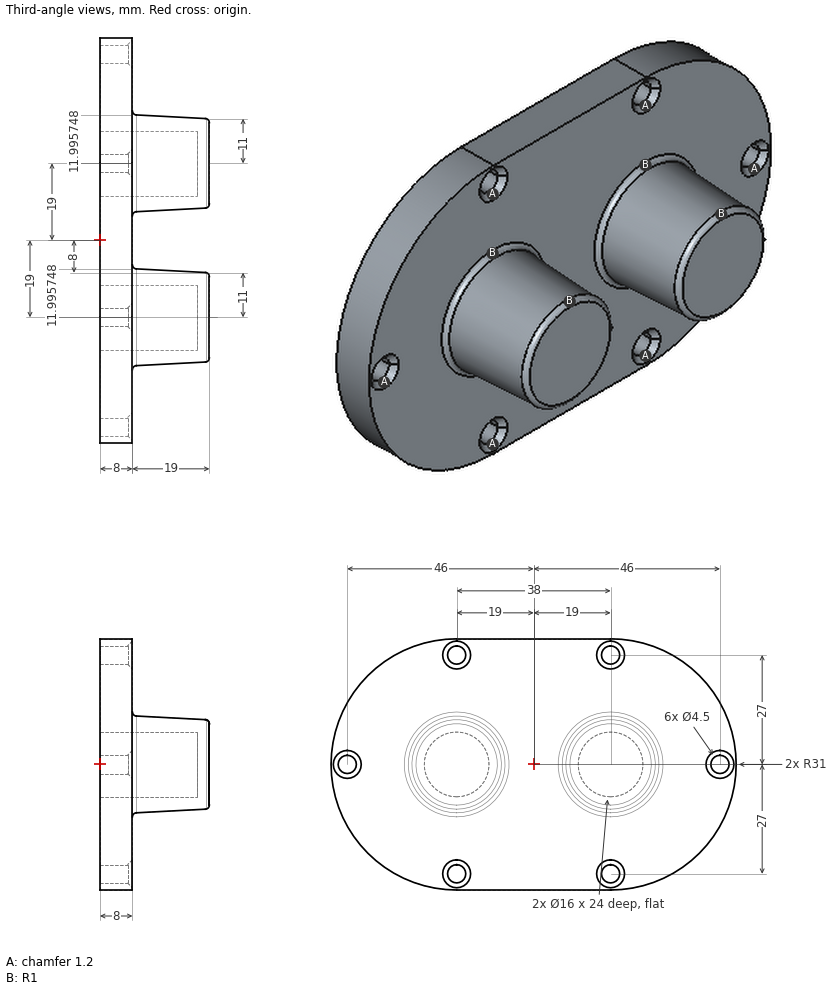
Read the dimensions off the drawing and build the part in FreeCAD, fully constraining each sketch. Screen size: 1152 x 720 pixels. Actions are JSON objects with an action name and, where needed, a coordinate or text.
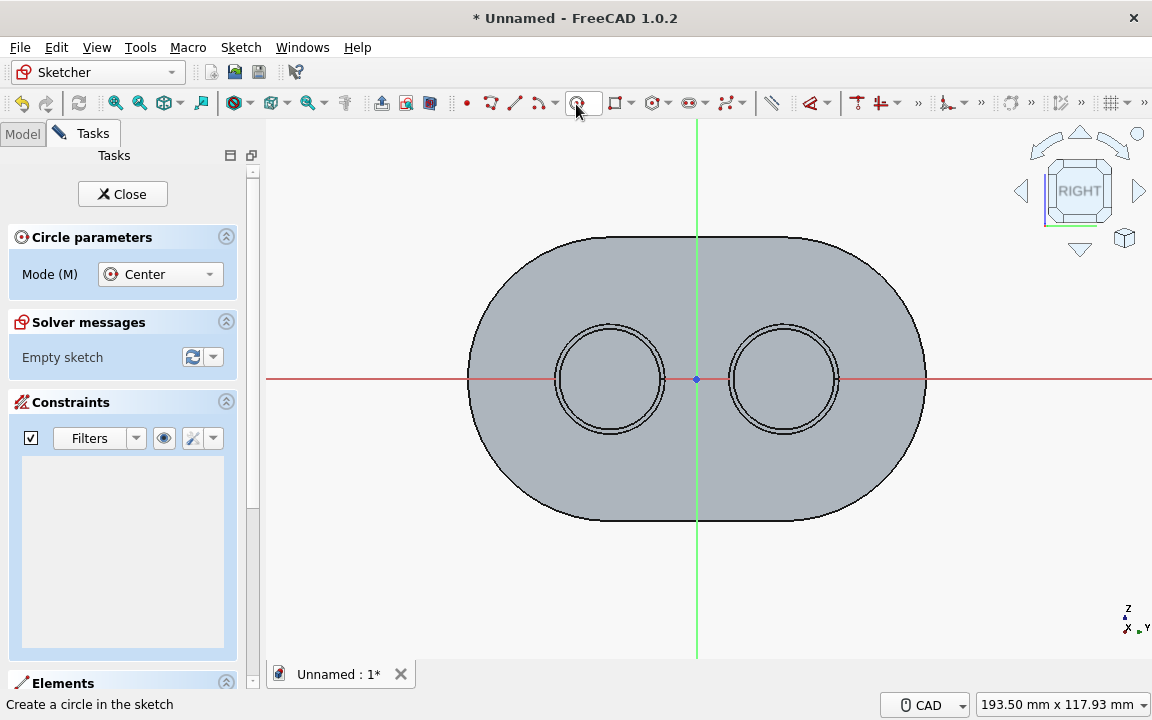
{"action": "scroll", "coordinate": [908, 379], "scroll_direction": "up", "scroll_amount": 4}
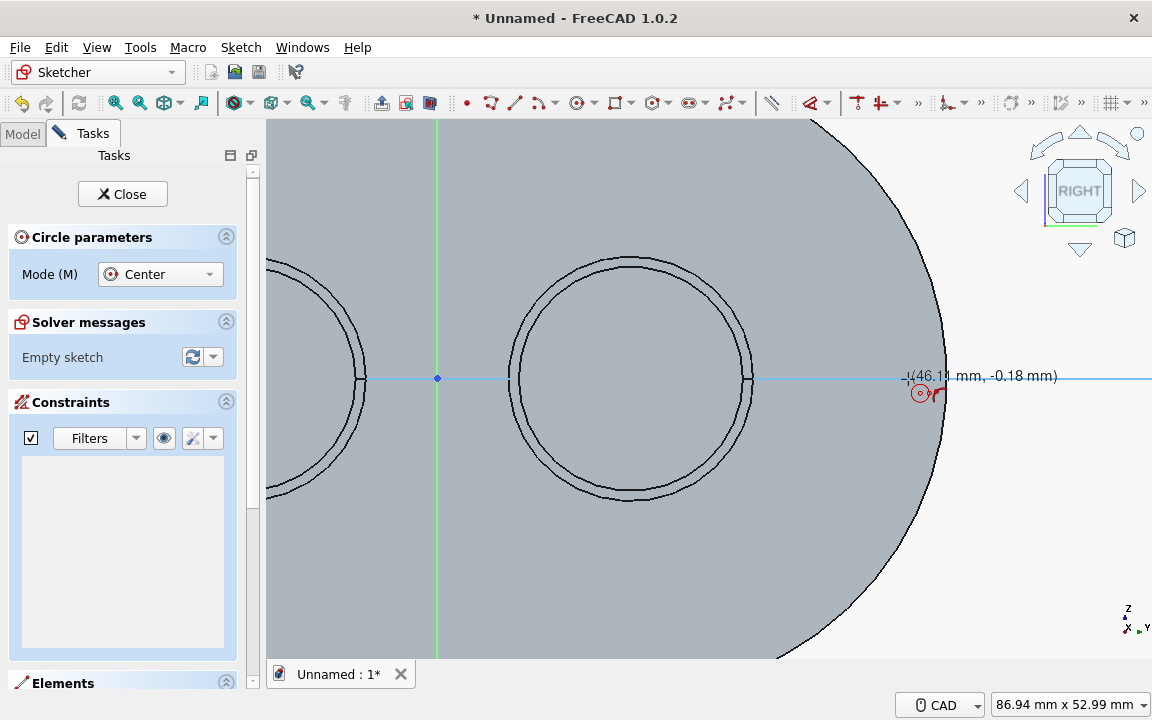
{"action": "left_click", "coordinate": [906, 379]}
{"action": "mouse_move", "coordinate": [922, 363]}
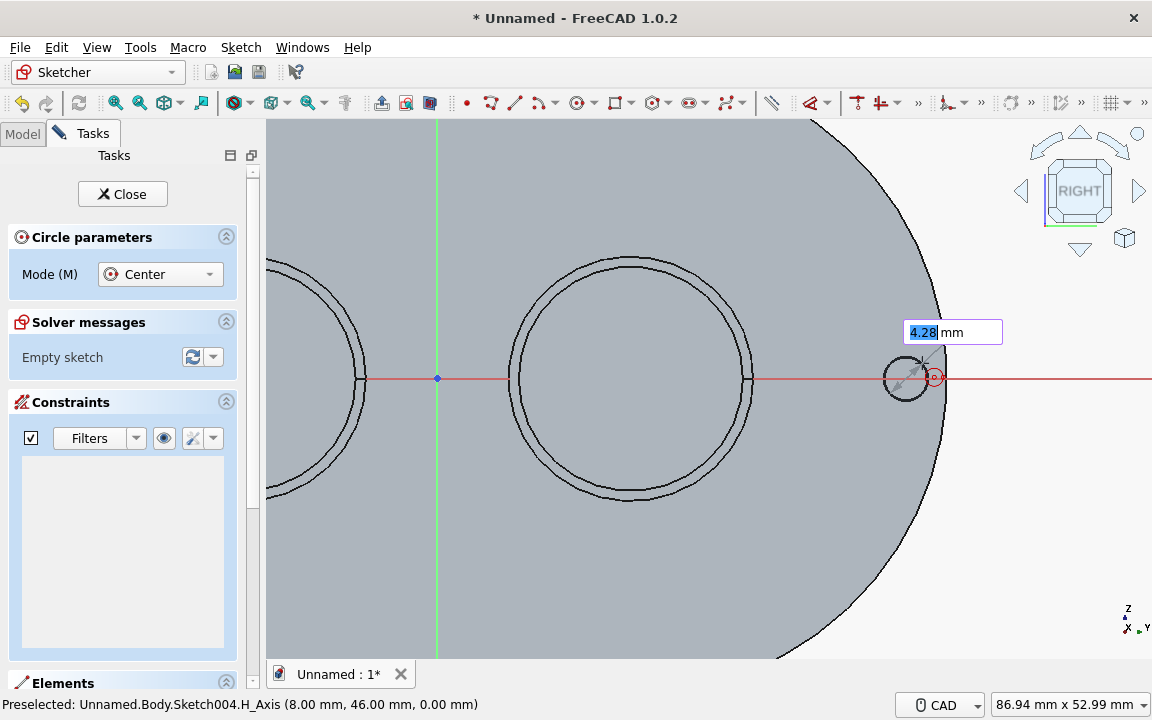
{"action": "type", "text": "4.5"}
{"action": "key", "text": "Return"}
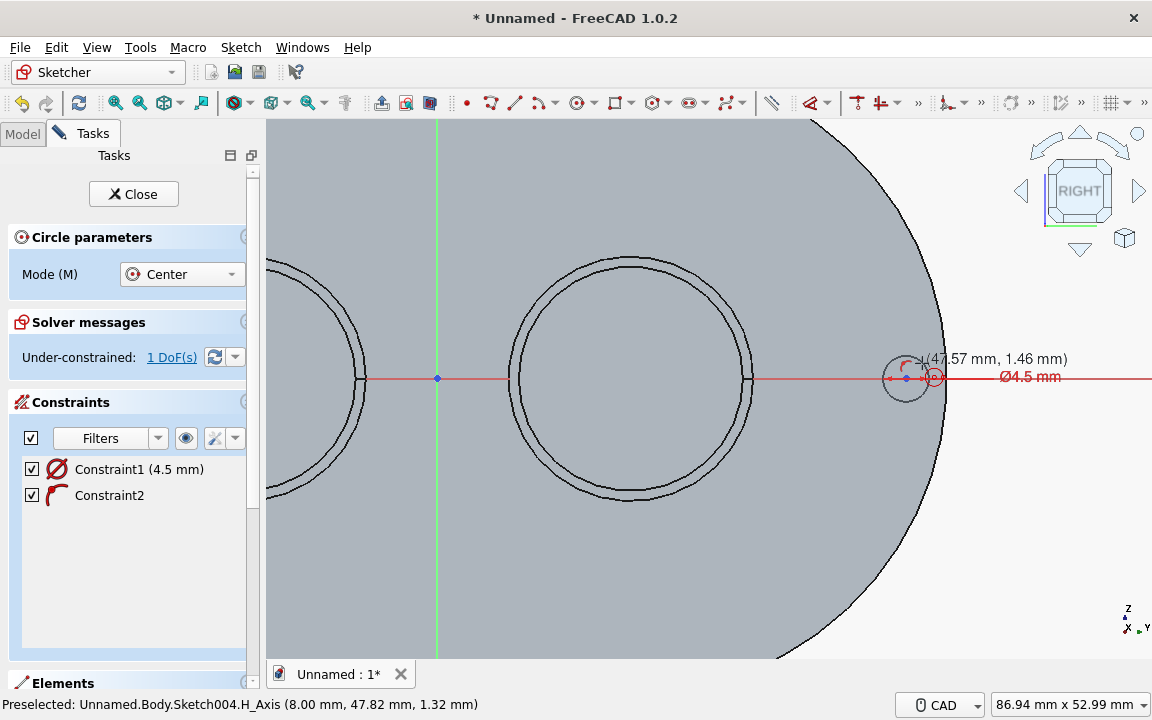
{"action": "scroll", "coordinate": [888, 401], "scroll_direction": "down", "scroll_amount": 3}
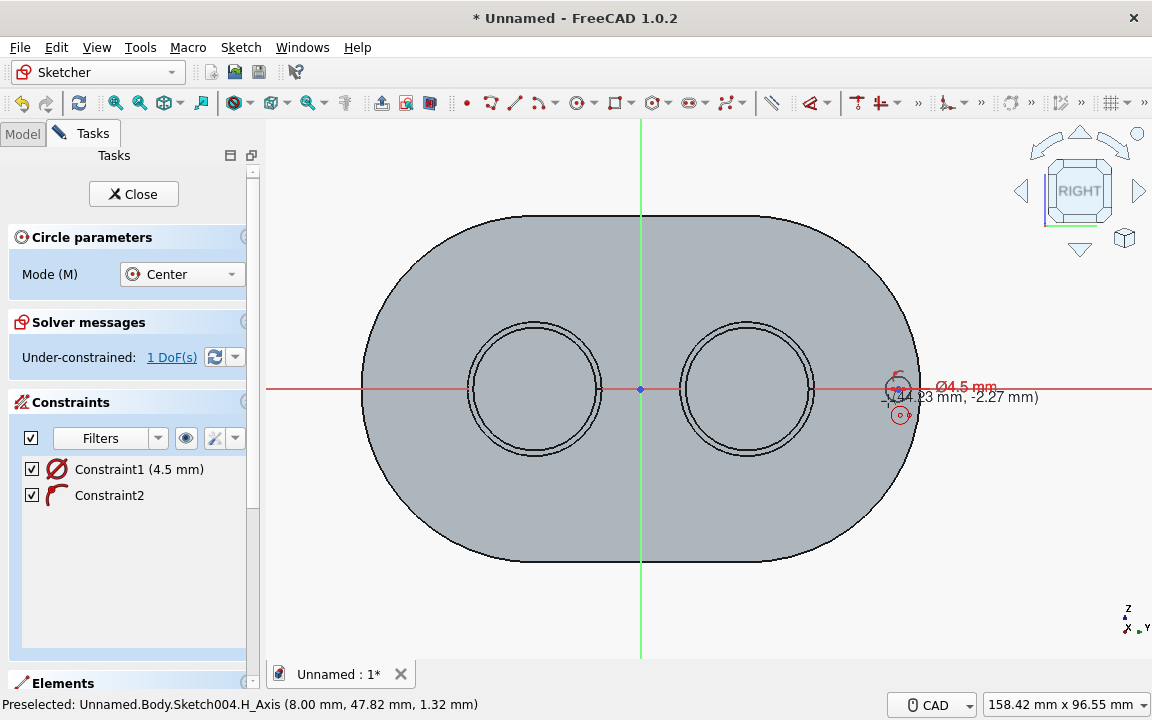
{"action": "scroll", "coordinate": [747, 238], "scroll_direction": "up", "scroll_amount": 3}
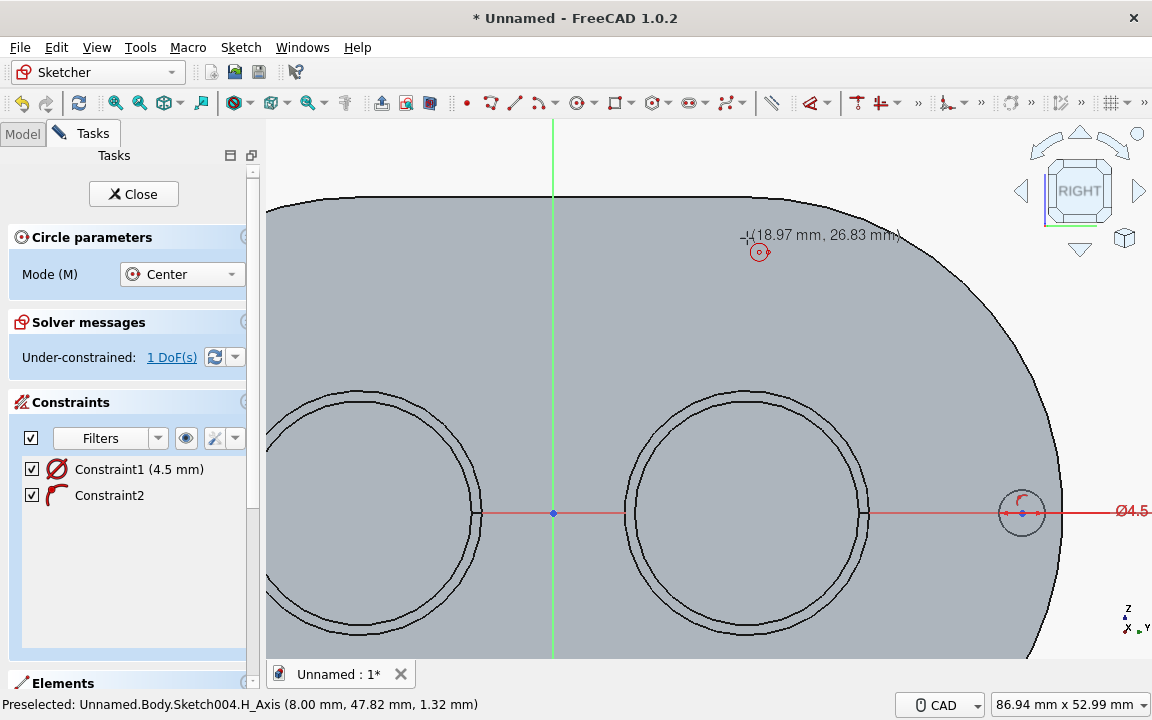
{"action": "left_click", "coordinate": [747, 238]}
{"action": "mouse_move", "coordinate": [763, 222]}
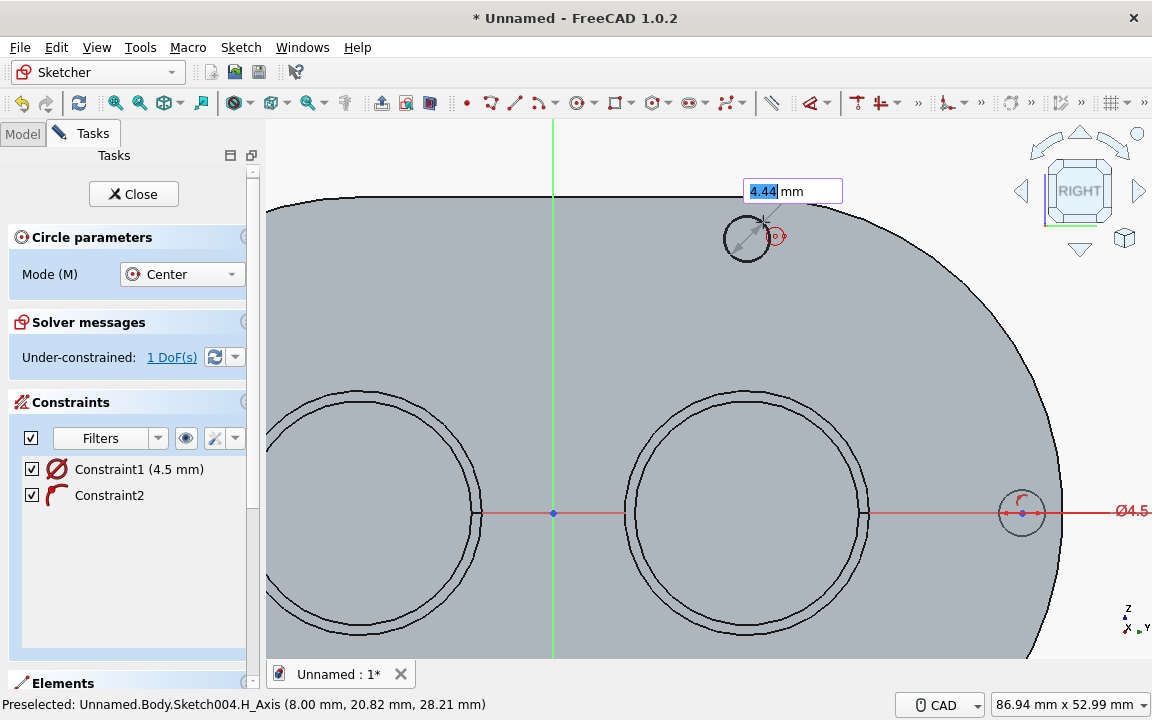
{"action": "type", "text": "4.5"}
{"action": "key", "text": "Return"}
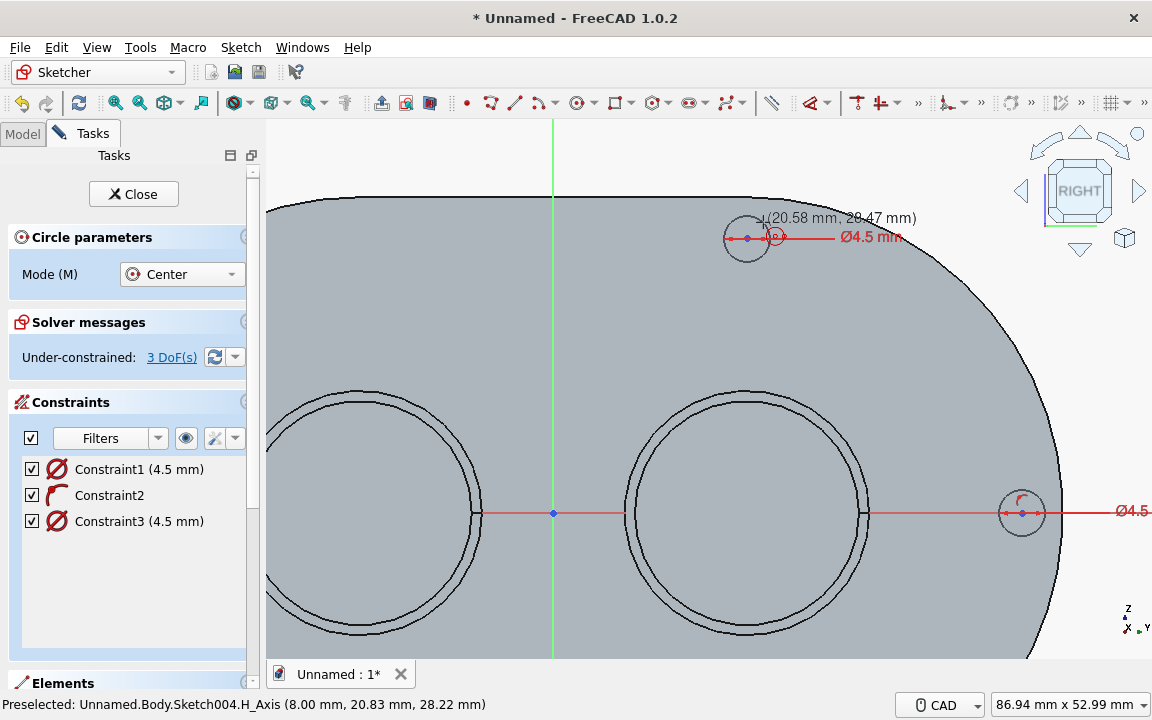
{"action": "scroll", "coordinate": [747, 238], "scroll_direction": "down", "scroll_amount": 3}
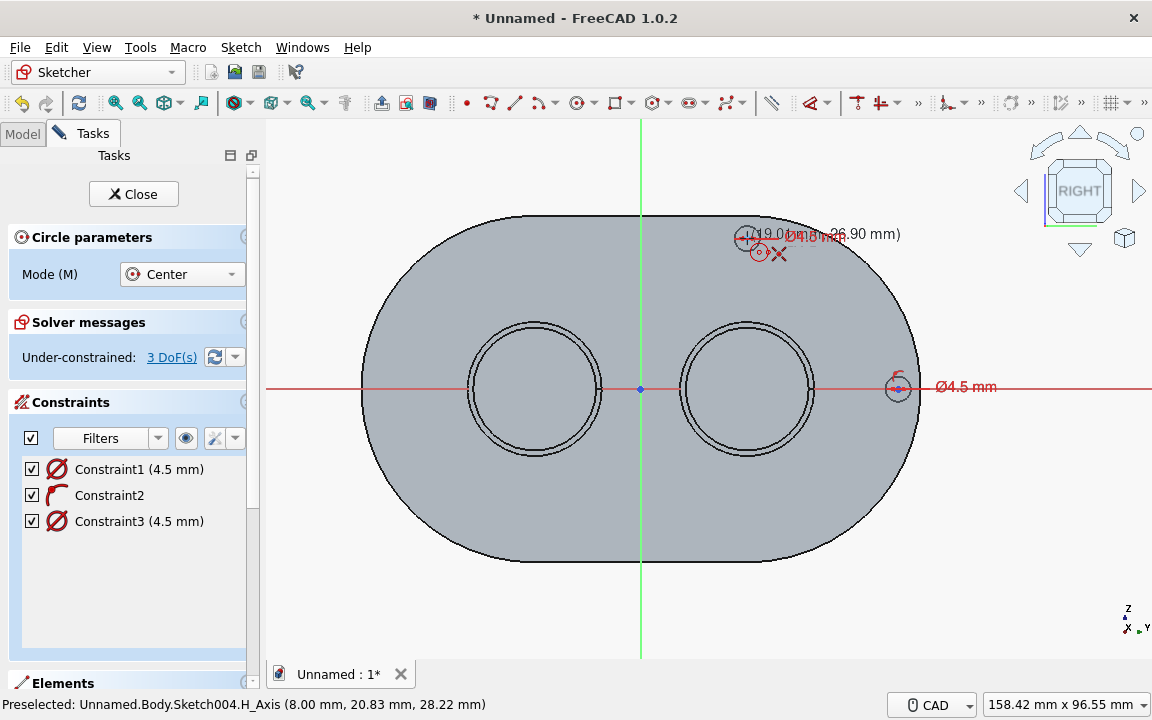
{"action": "scroll", "coordinate": [747, 540], "scroll_direction": "up", "scroll_amount": 3}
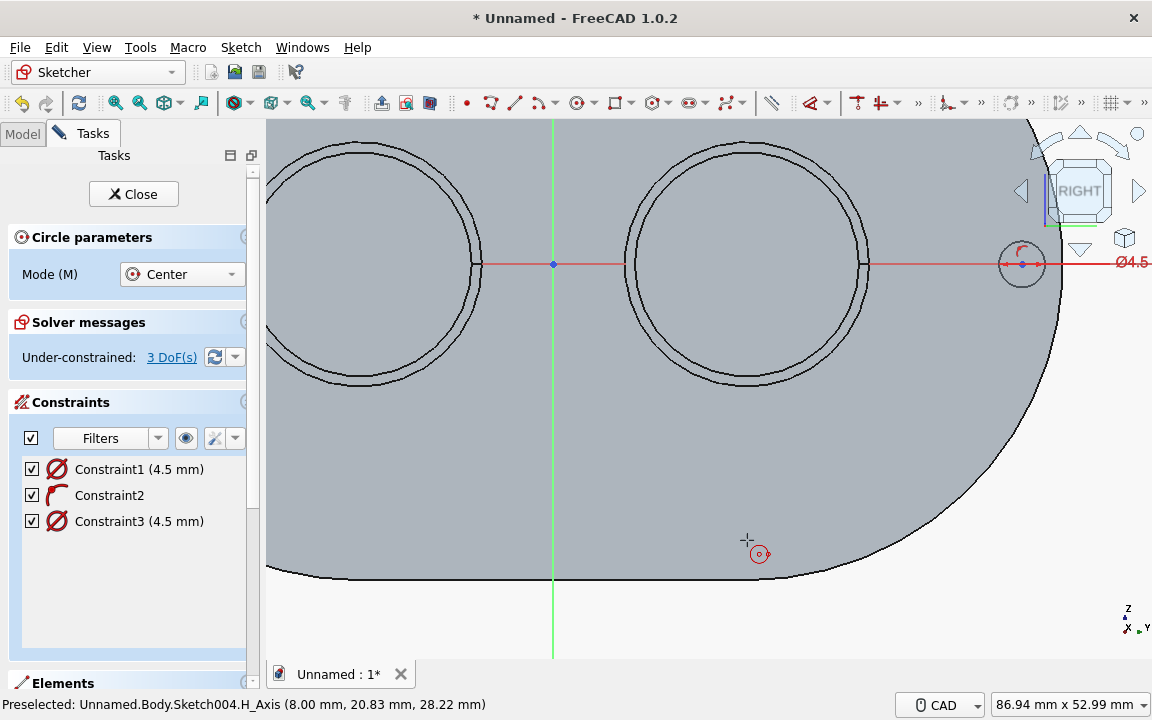
{"action": "left_click", "coordinate": [747, 539]}
{"action": "mouse_move", "coordinate": [763, 523]}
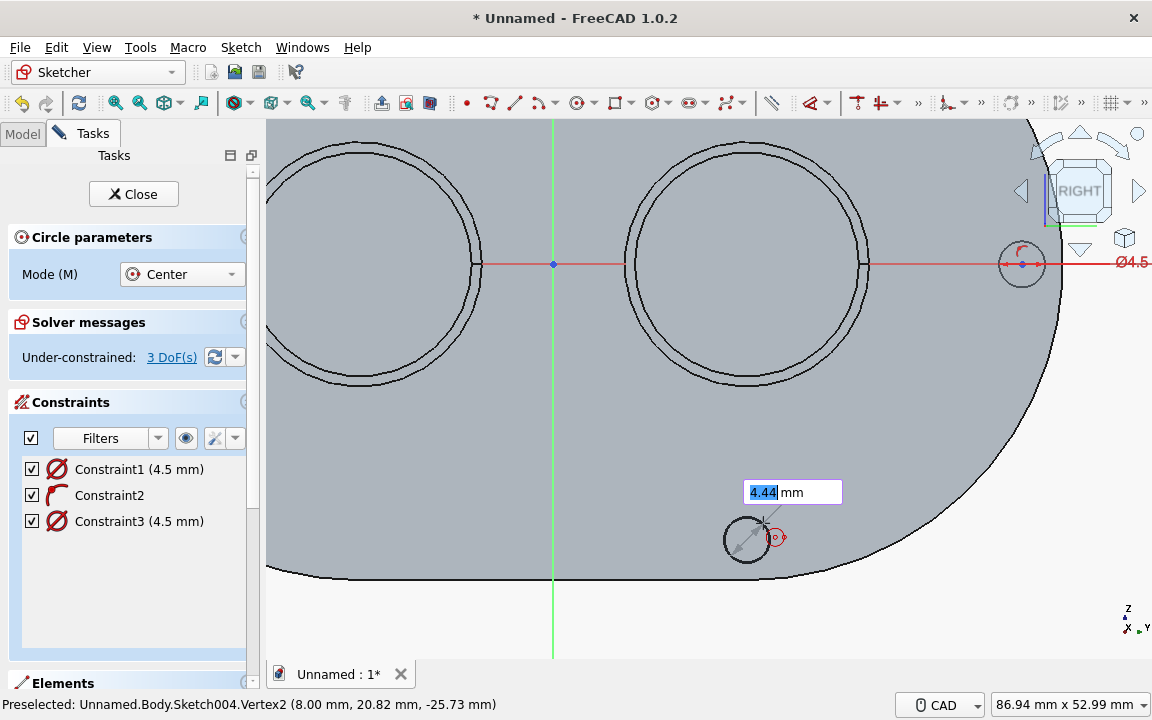
{"action": "type", "text": "4.5"}
{"action": "key", "text": "Return"}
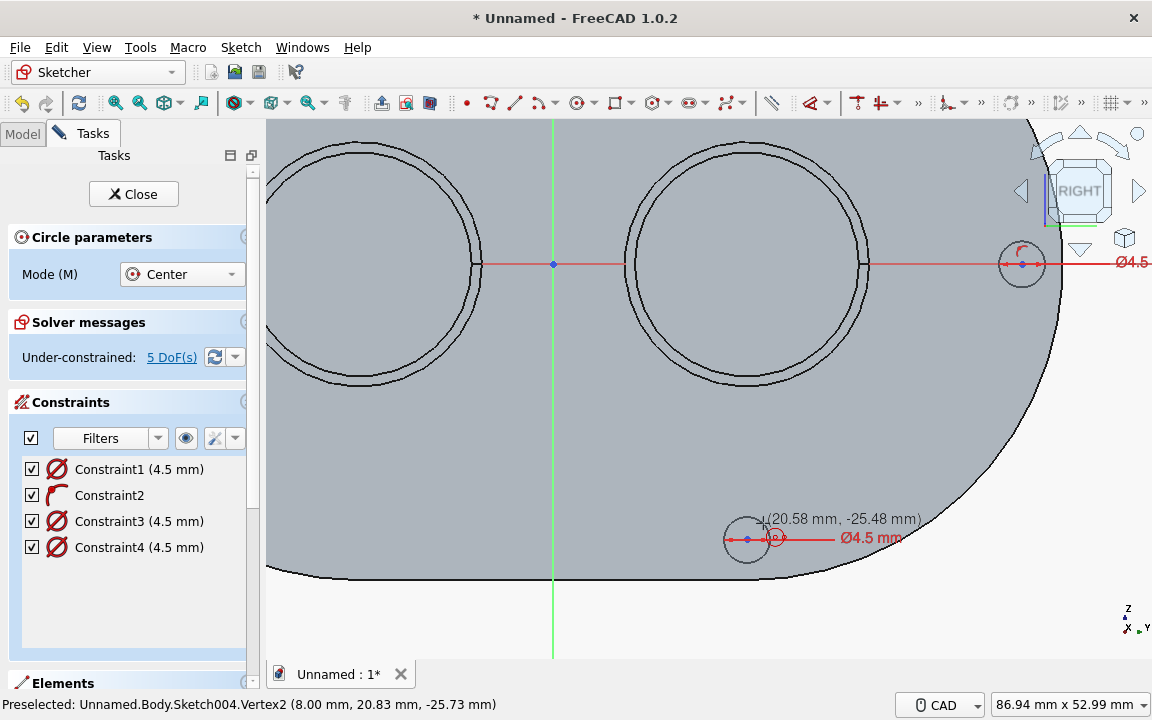
{"action": "scroll", "coordinate": [747, 541], "scroll_direction": "down", "scroll_amount": 3}